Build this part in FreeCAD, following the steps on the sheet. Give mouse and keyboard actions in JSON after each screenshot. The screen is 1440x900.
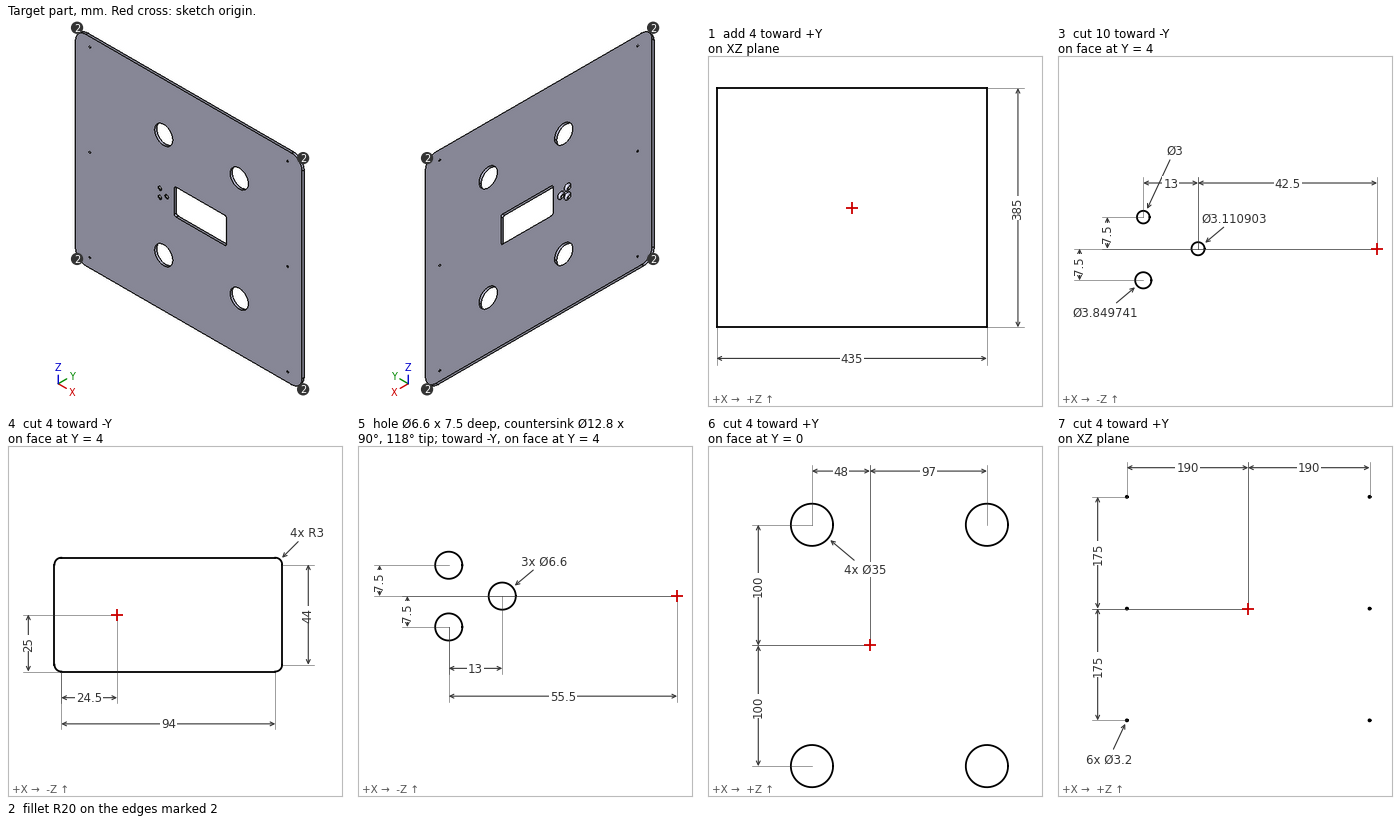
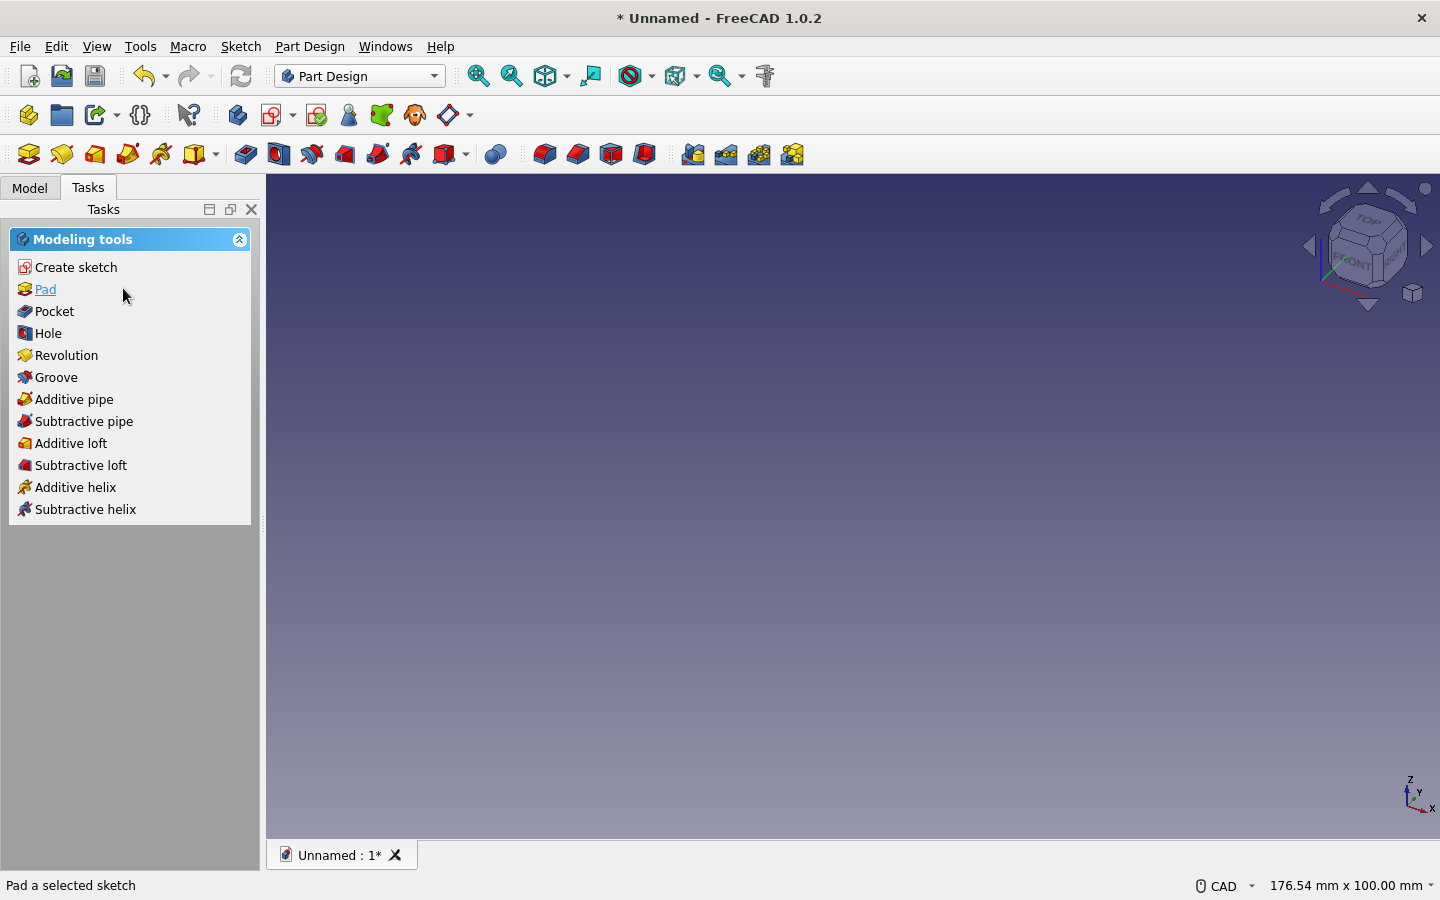
{"action": "left_click", "coordinate": [29, 154]}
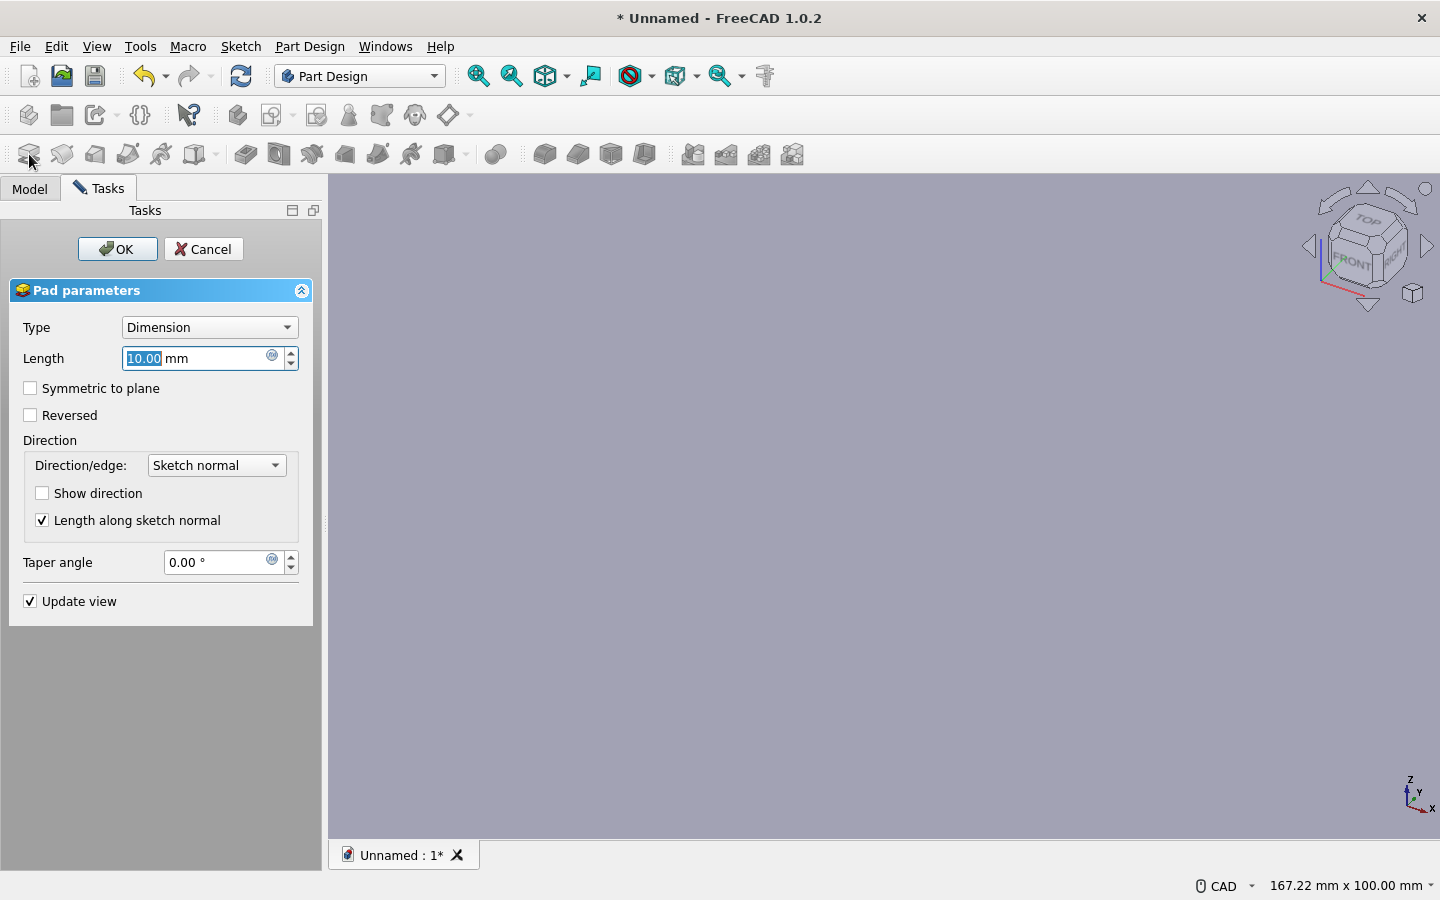
{"action": "type", "text": "4"}
{"action": "key", "text": "Tab"}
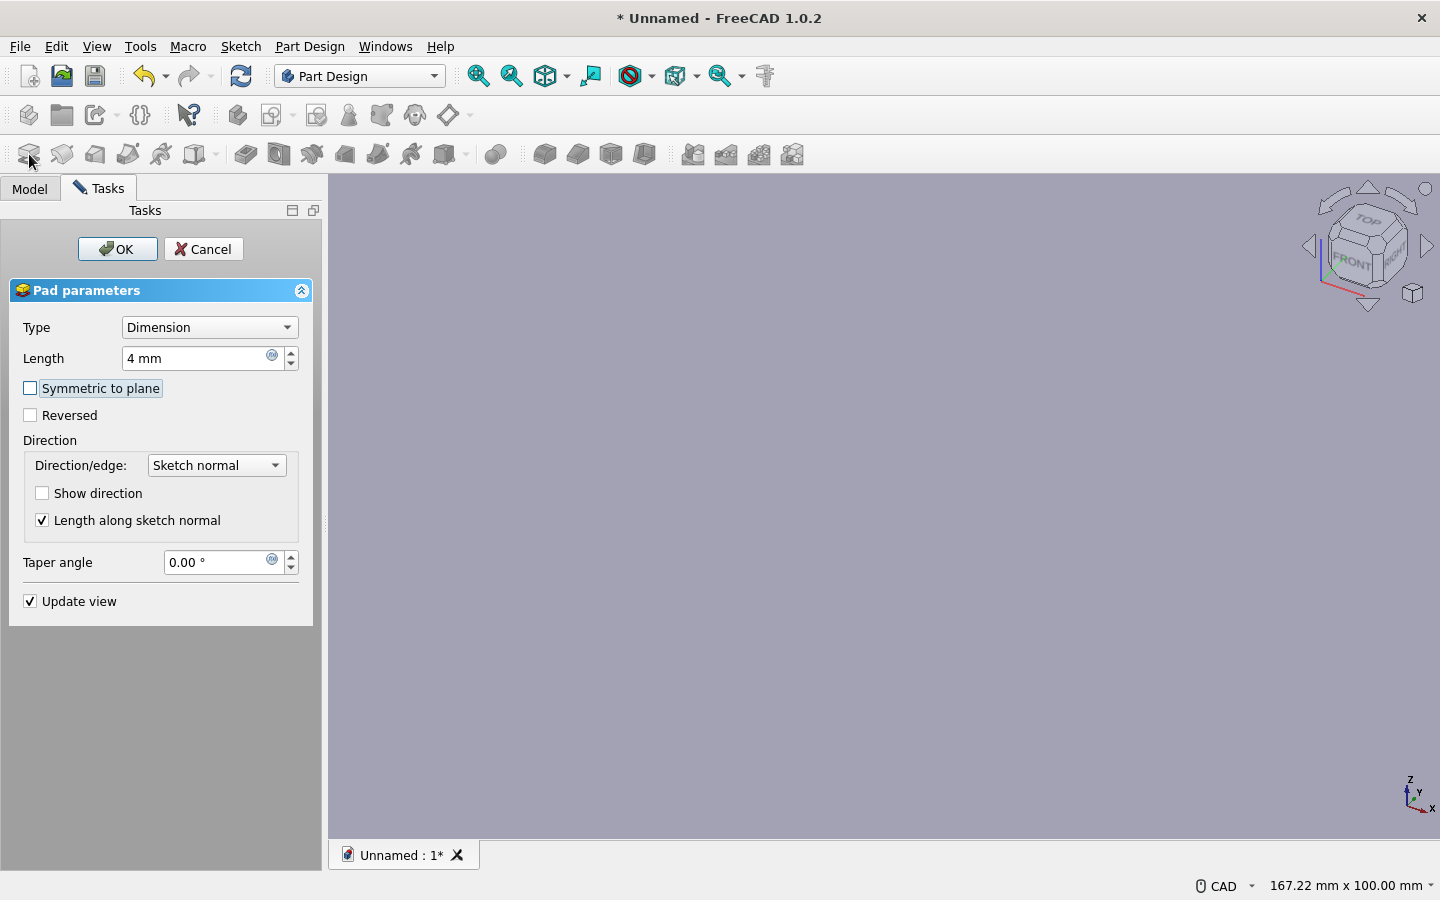
{"action": "left_click", "coordinate": [31, 415]}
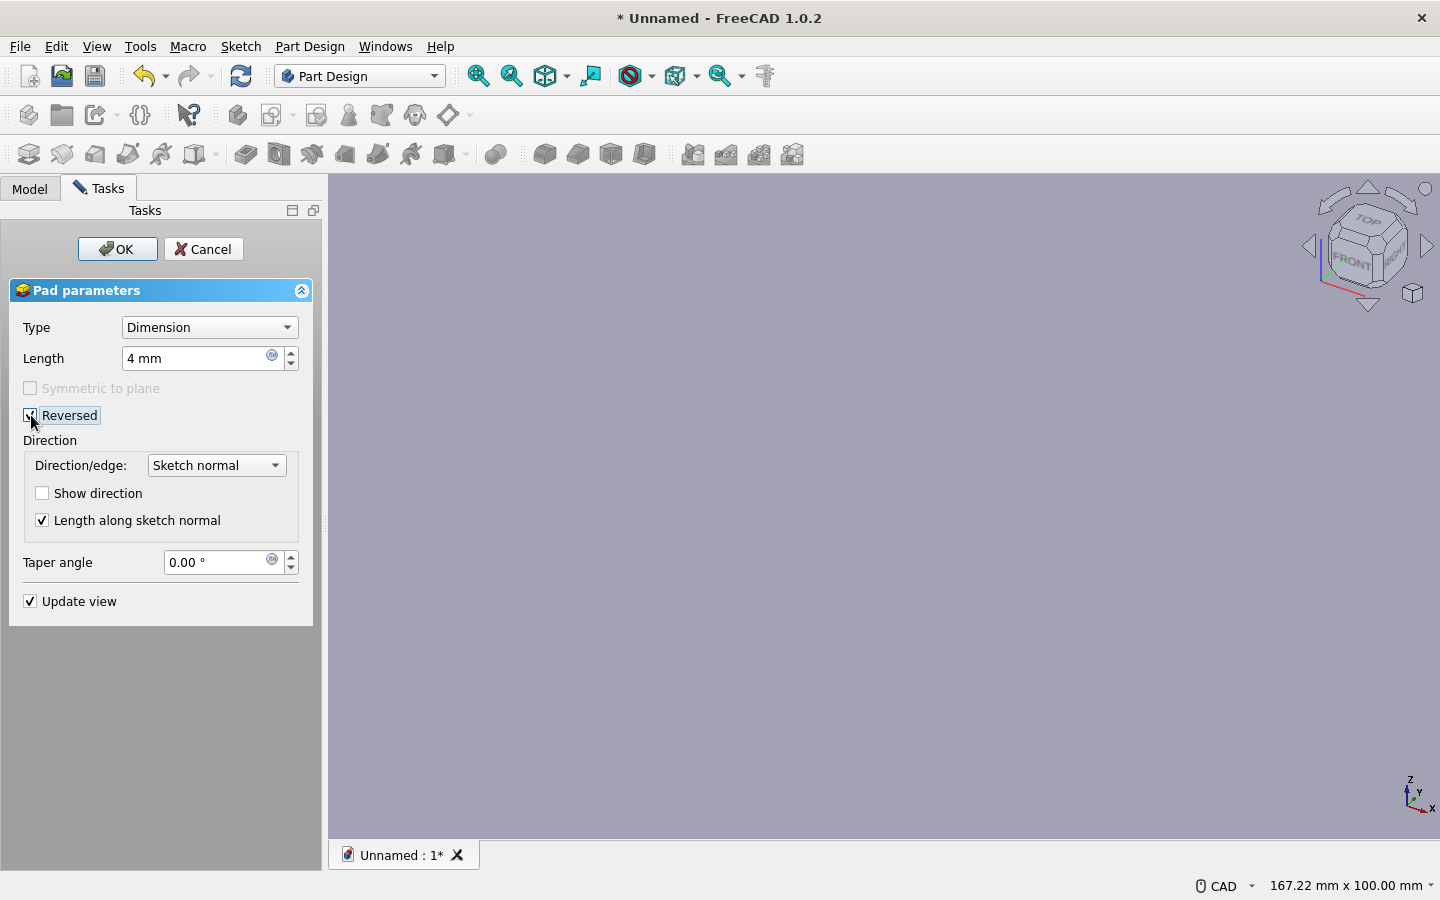
{"action": "left_click", "coordinate": [118, 249]}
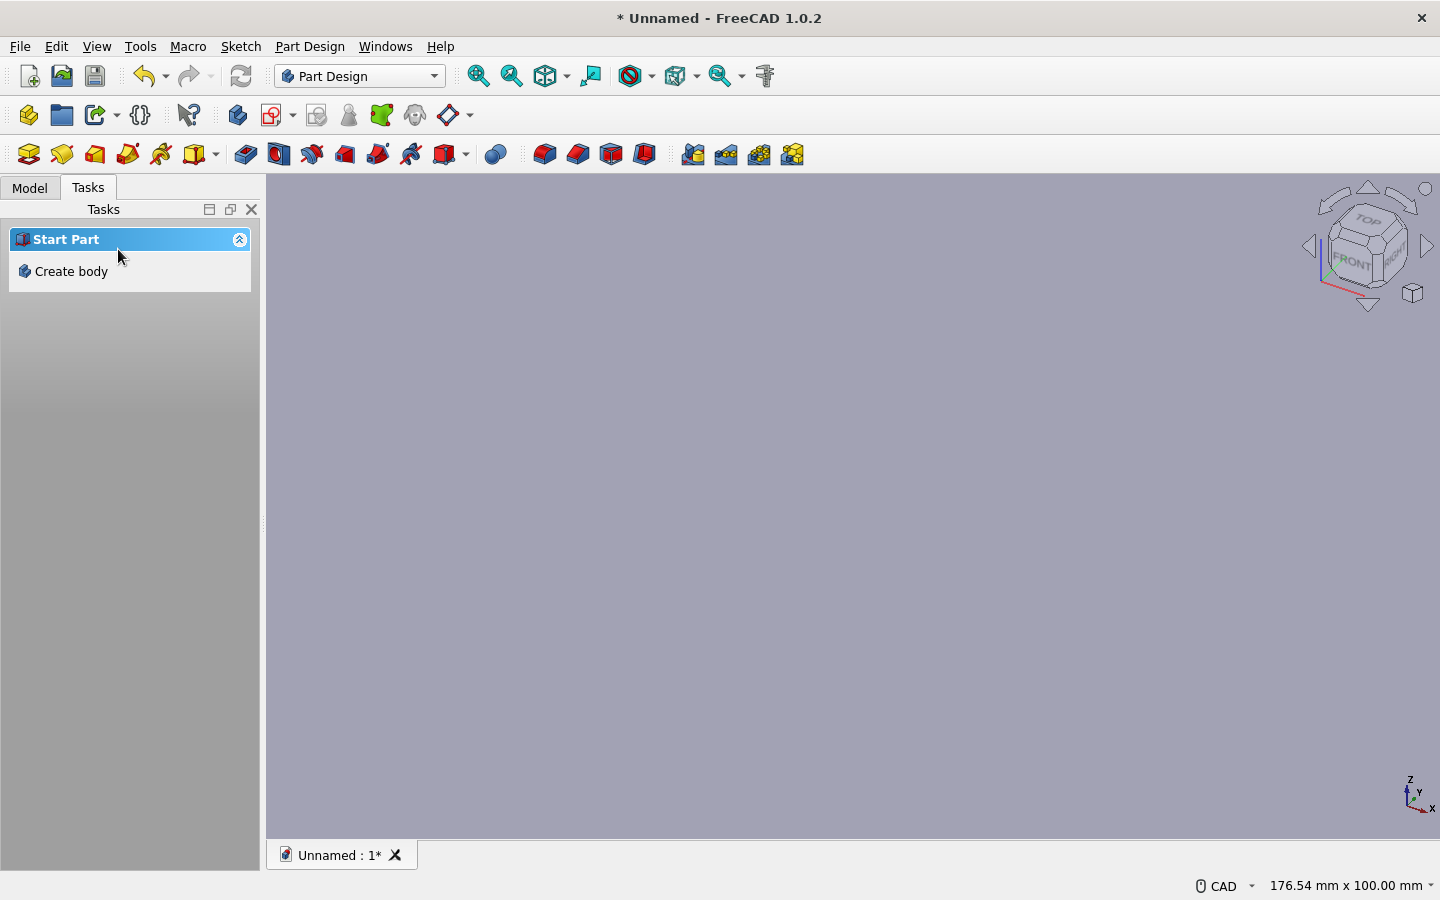
{"action": "left_click", "coordinate": [479, 76]}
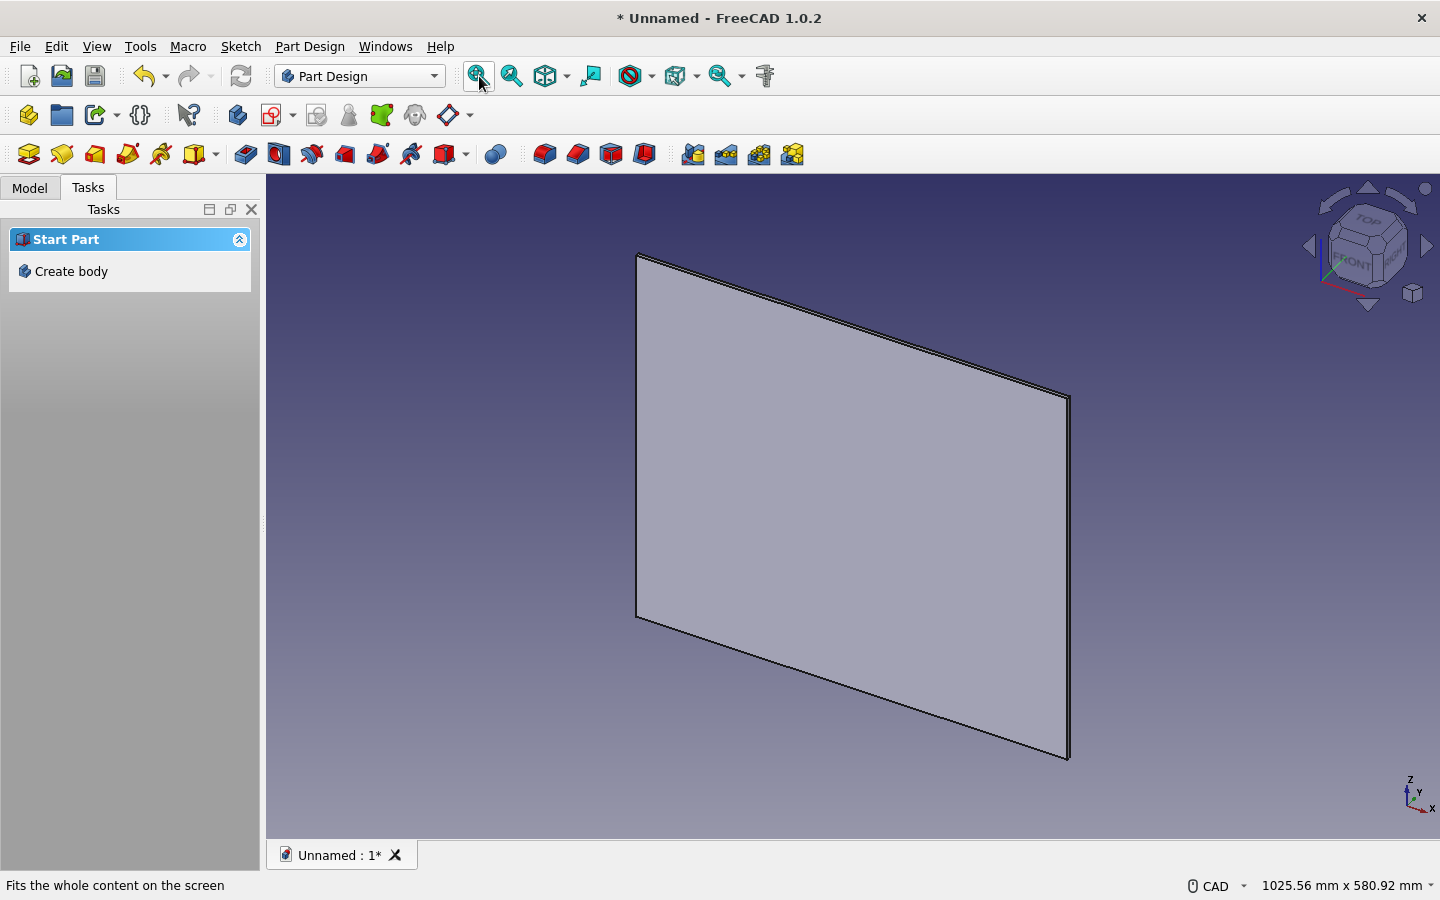
{"action": "scroll", "coordinate": [1069, 396], "scroll_direction": "up", "scroll_amount": 11}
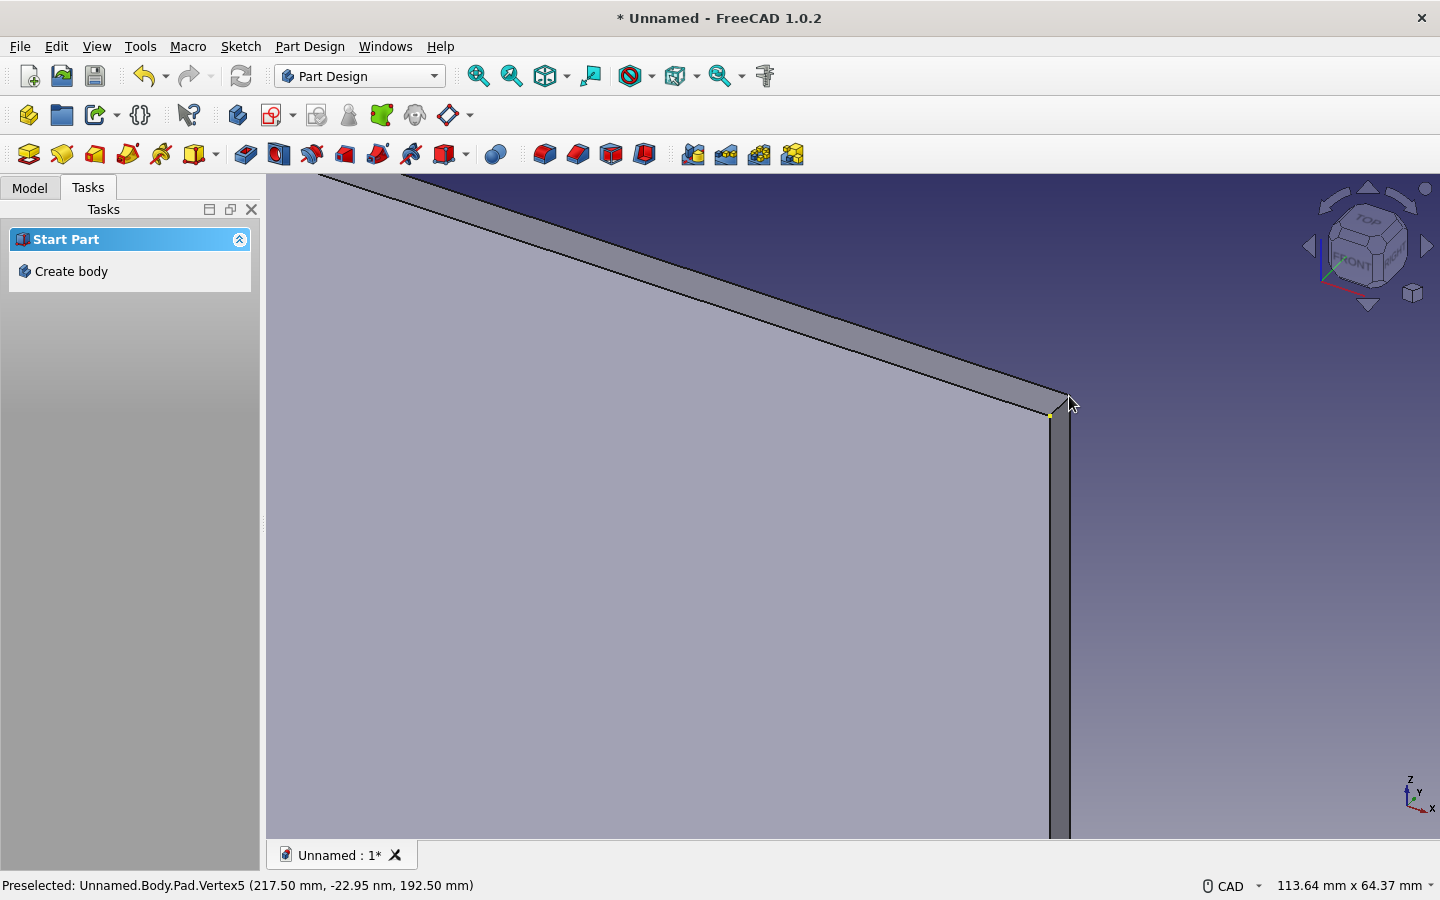
{"action": "left_click", "coordinate": [1060, 405]}